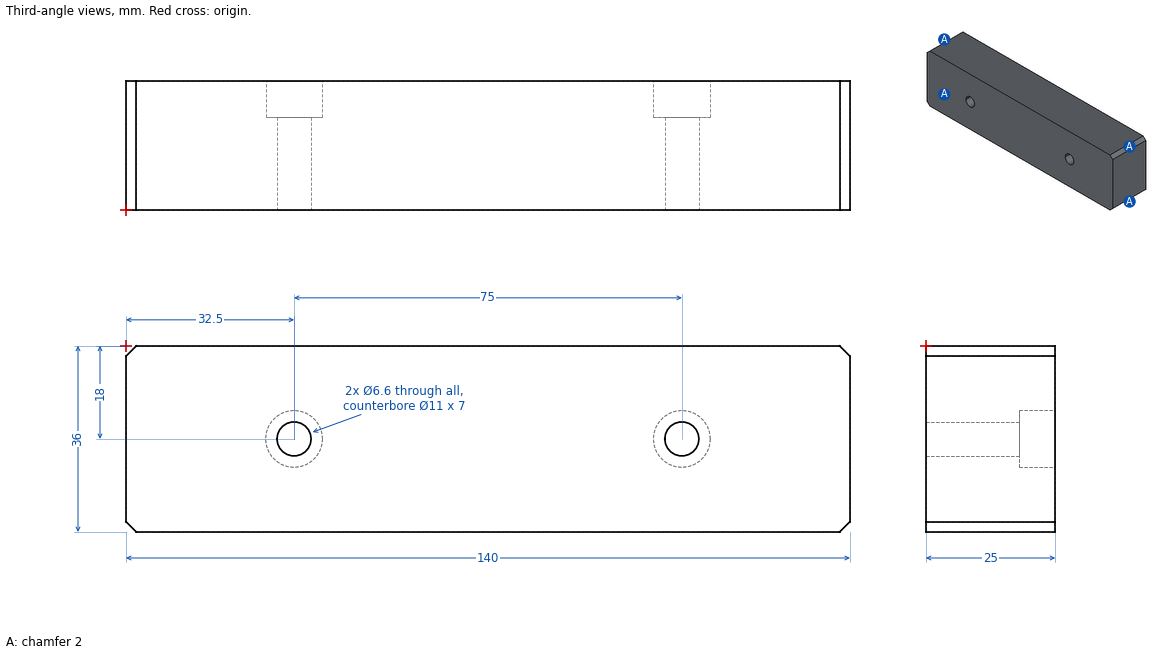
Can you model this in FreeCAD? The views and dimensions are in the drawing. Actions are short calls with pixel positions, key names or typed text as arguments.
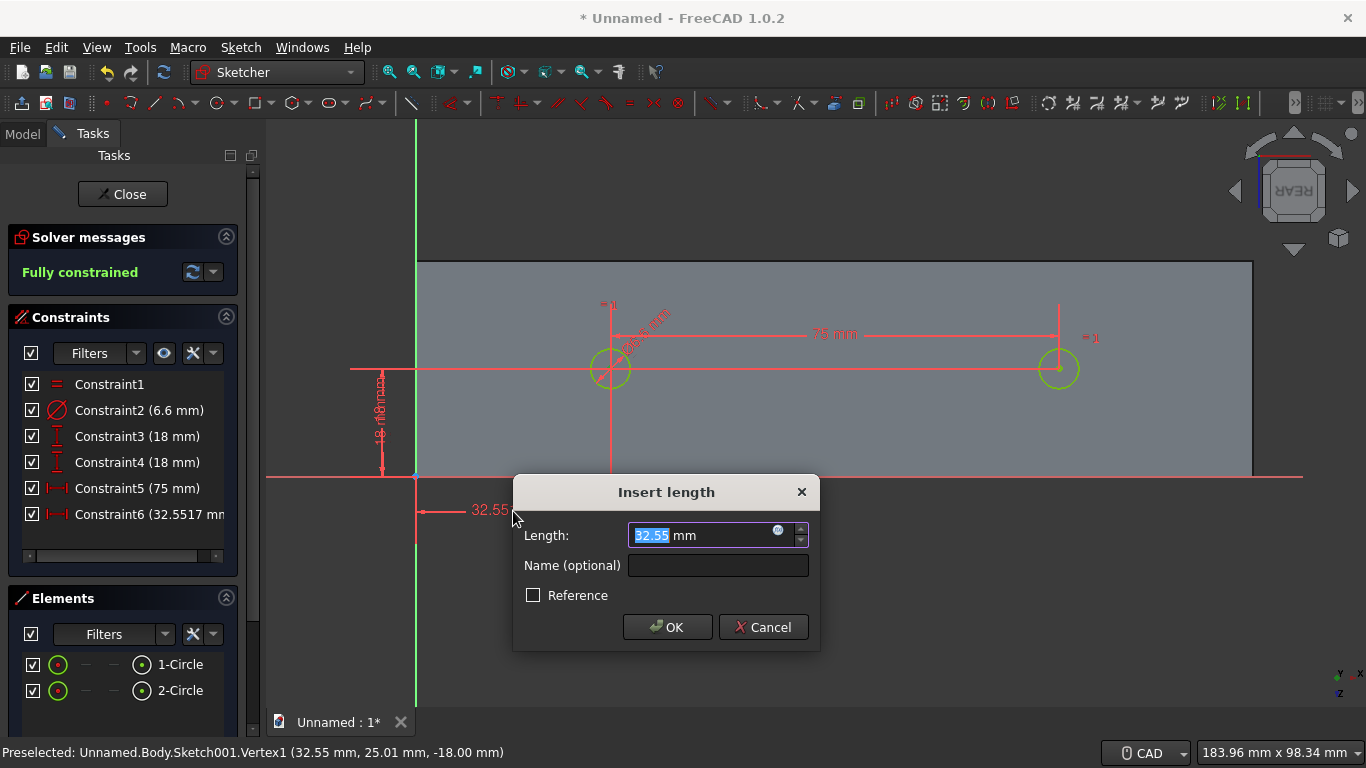
text(32.5)
key(Return)
key(Escape)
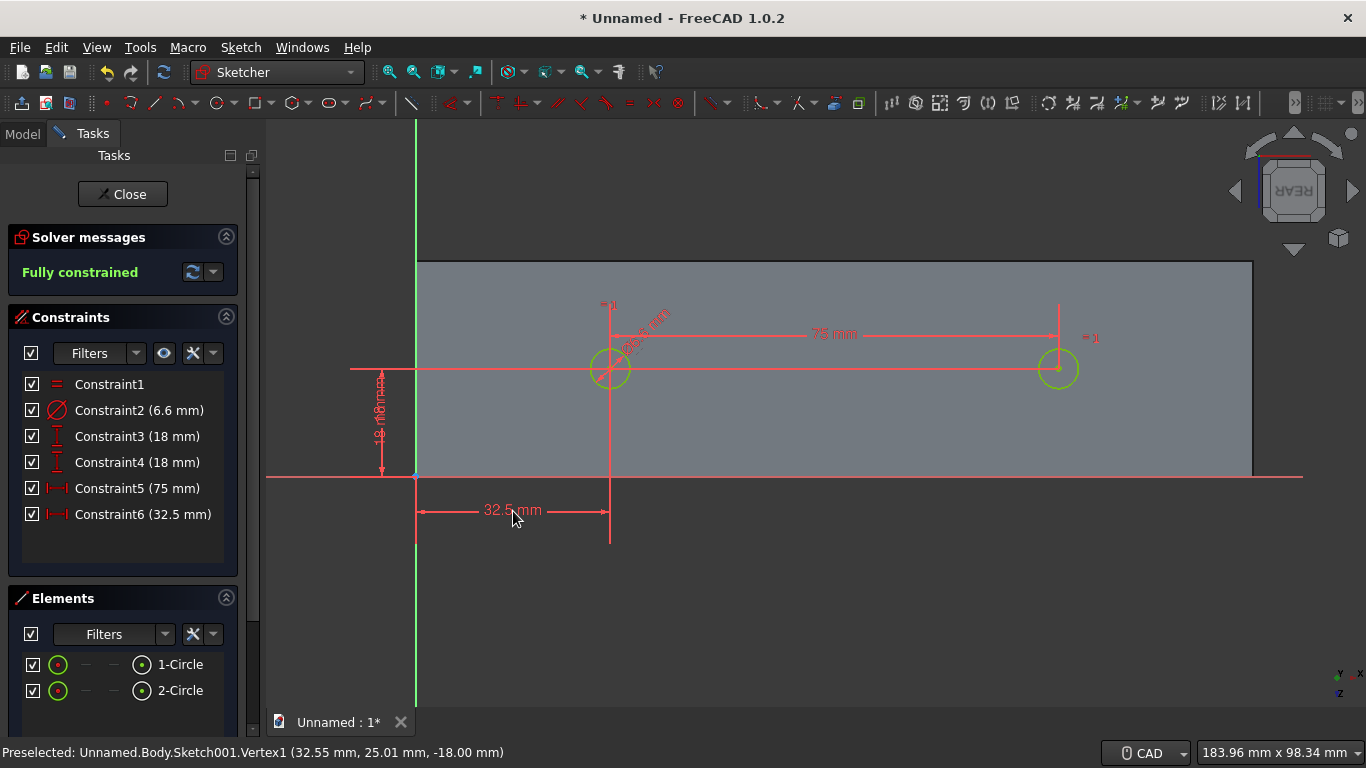
click(123, 194)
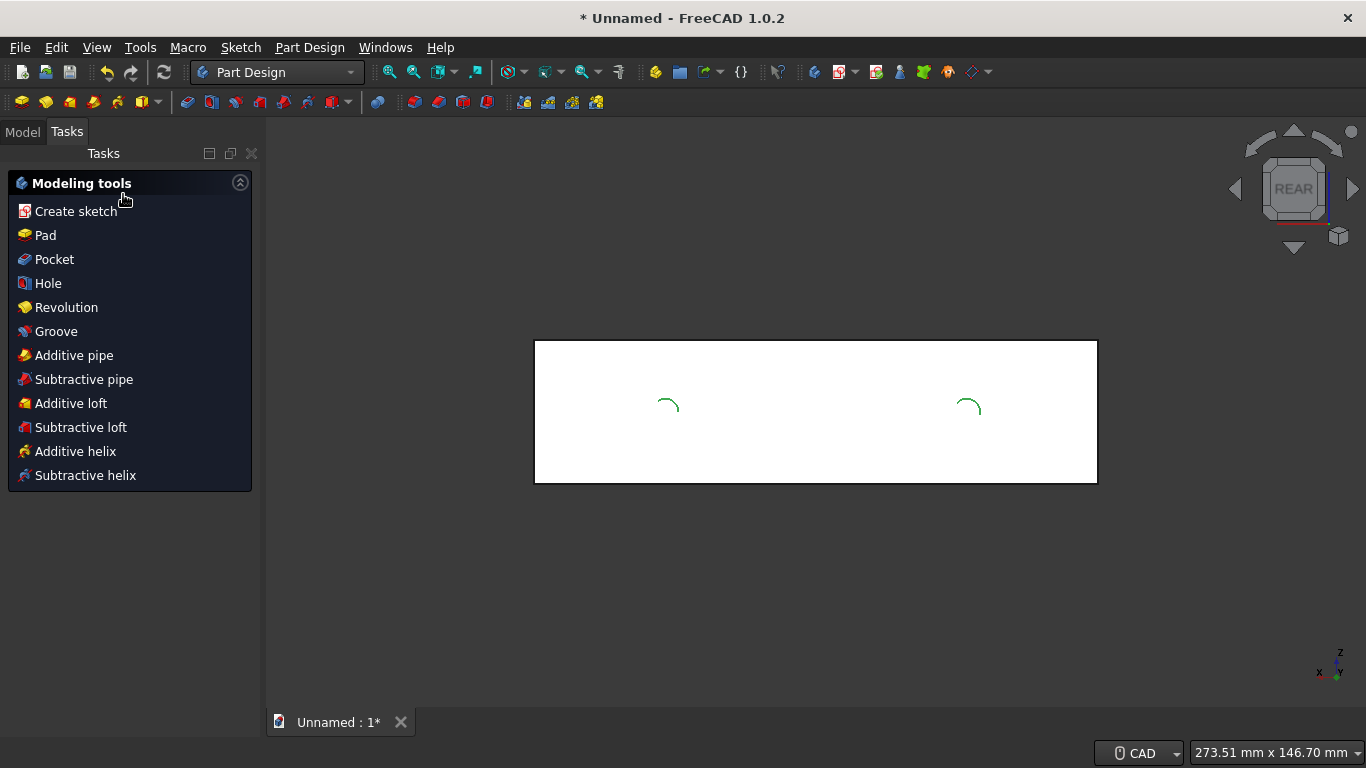
click(212, 102)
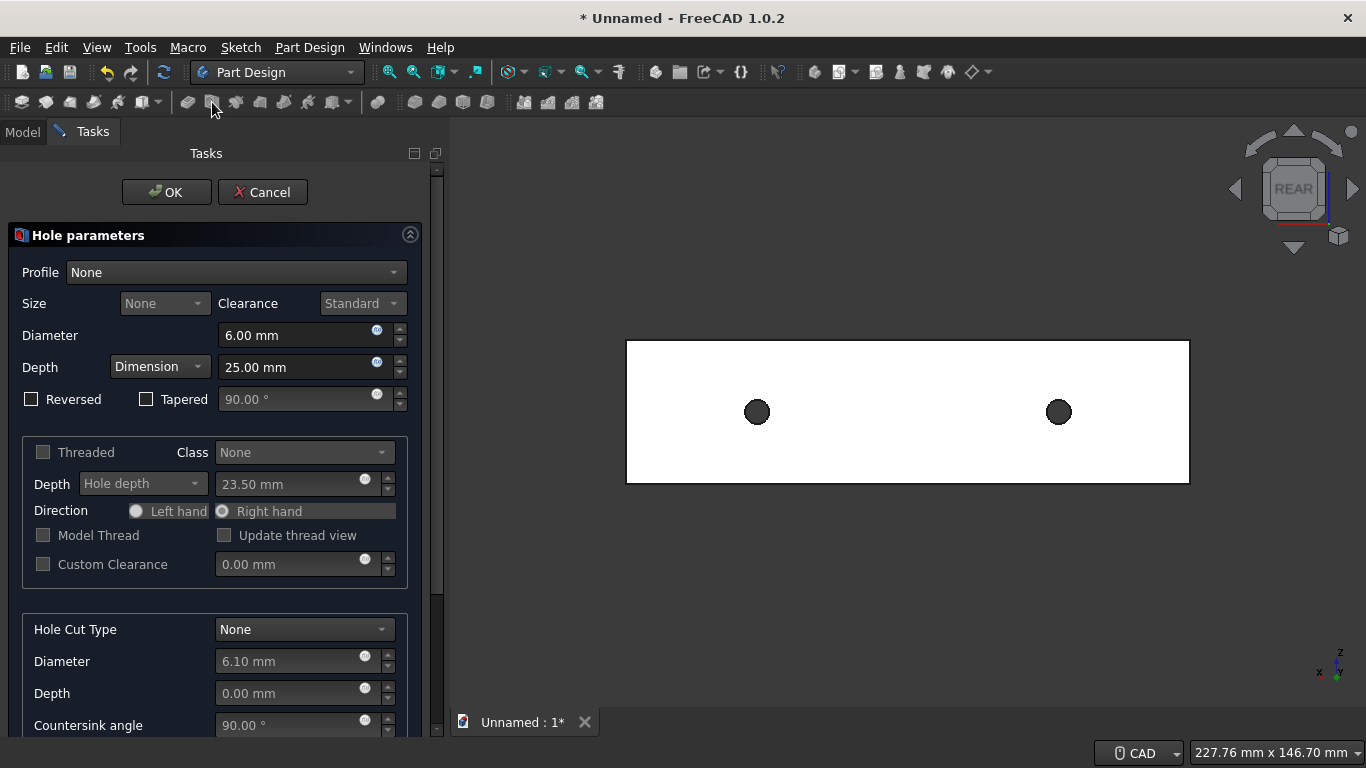
triple_click(305, 335)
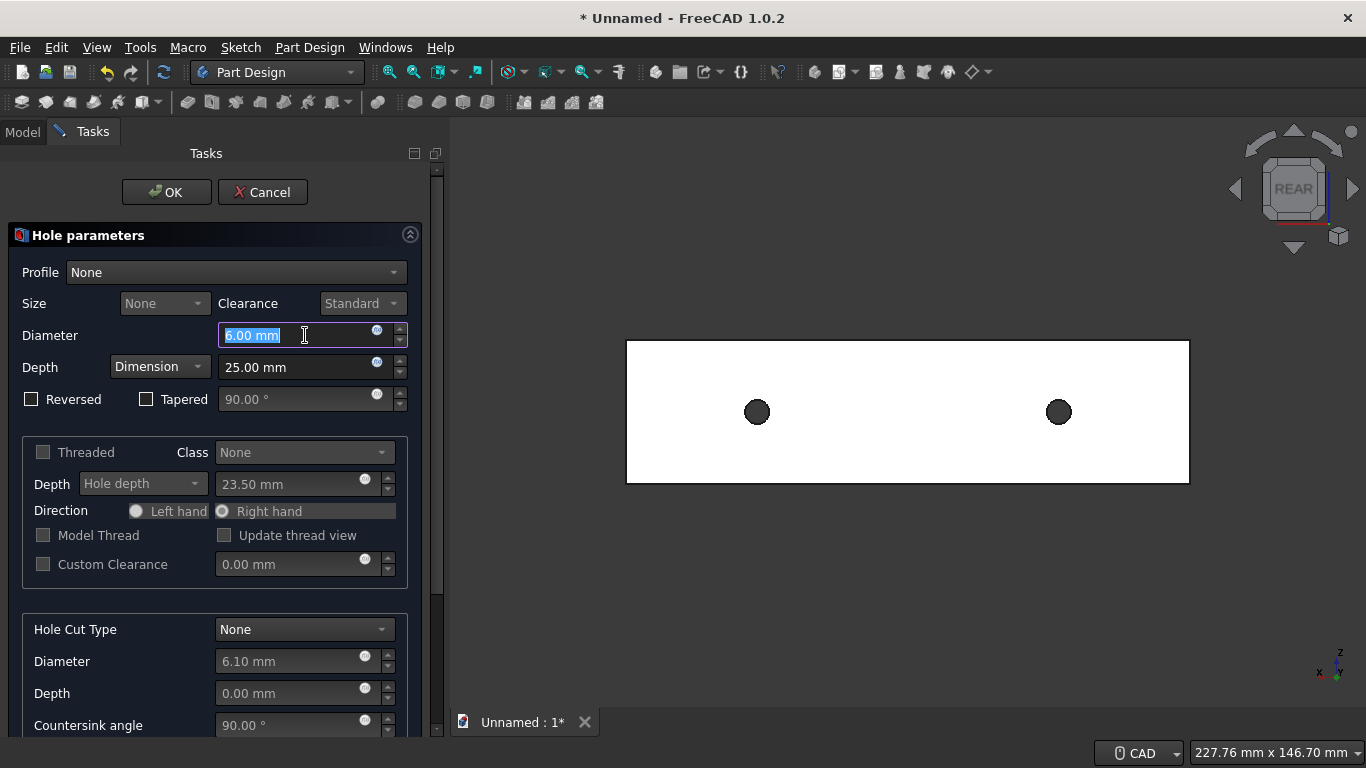
text(6.6)
key(Tab)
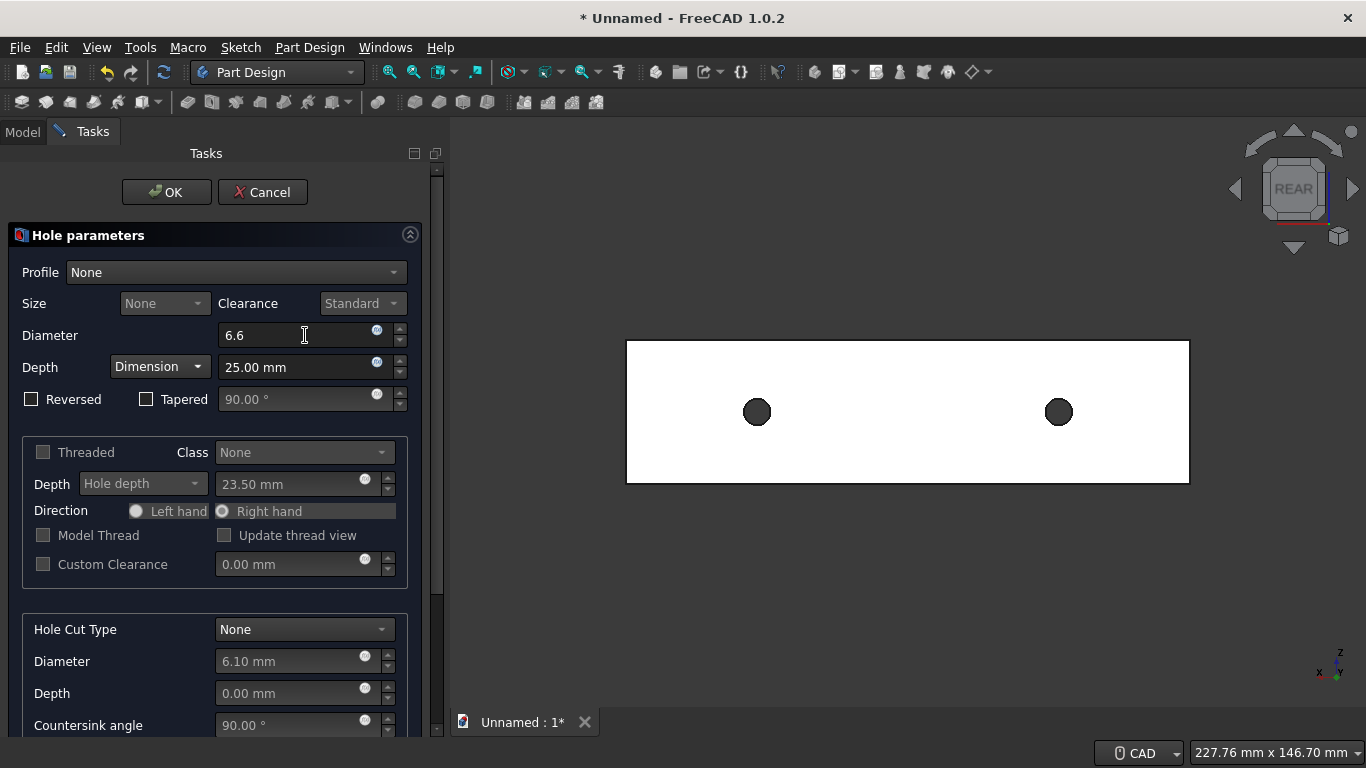
click(161, 366)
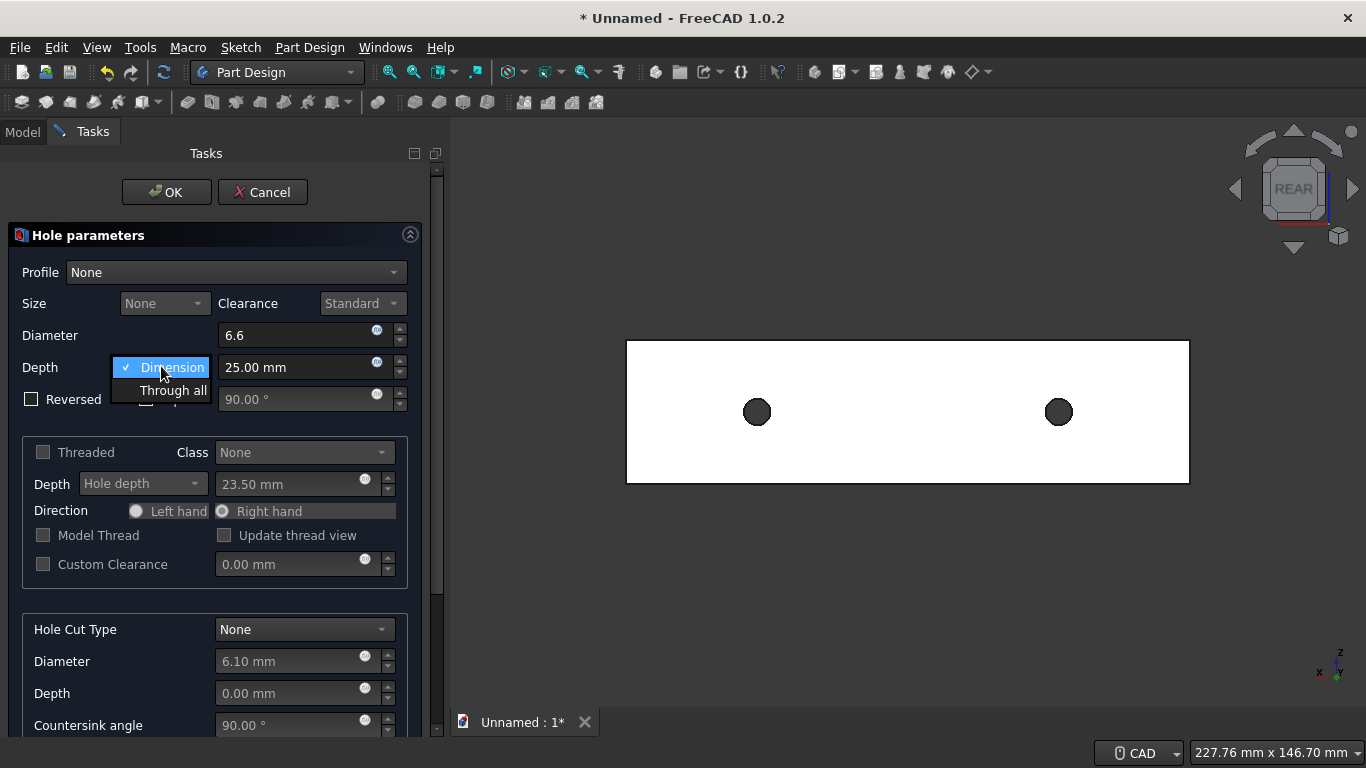
click(160, 390)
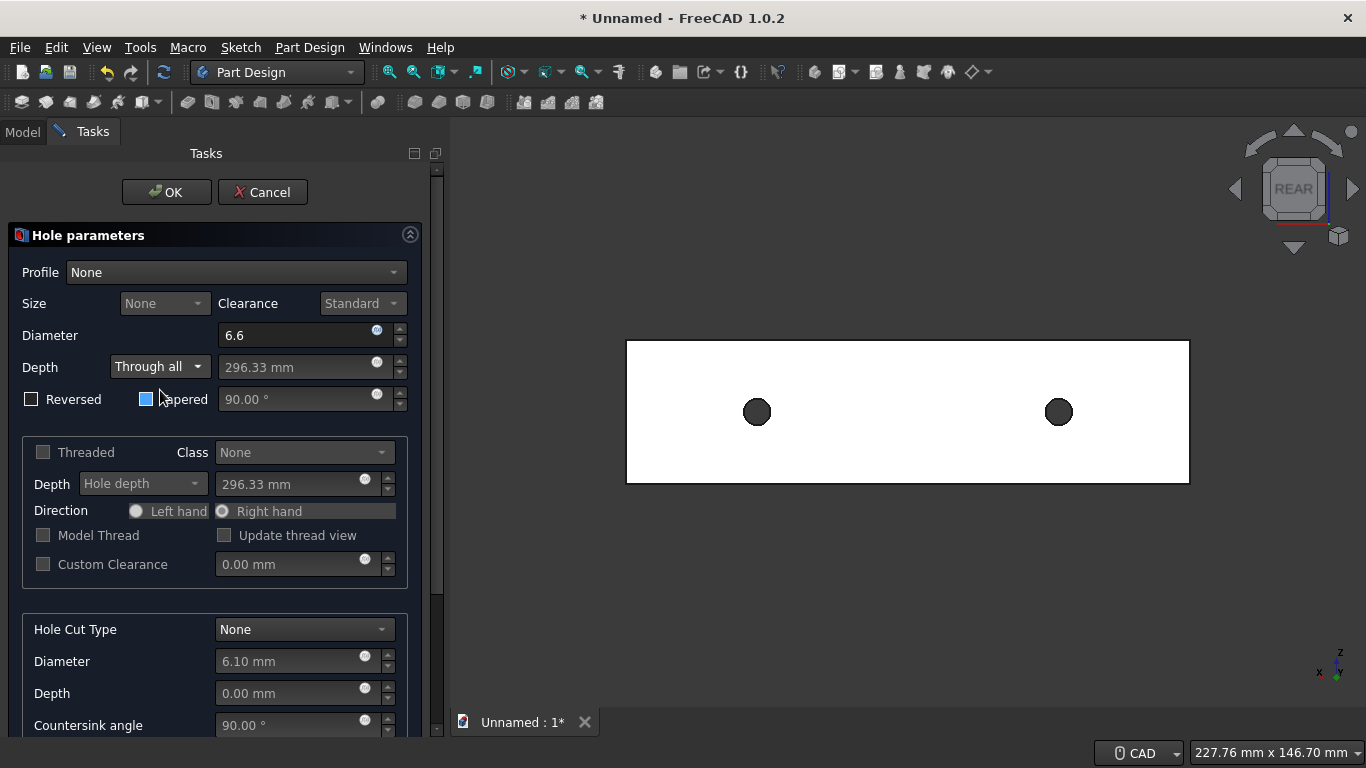
click(306, 630)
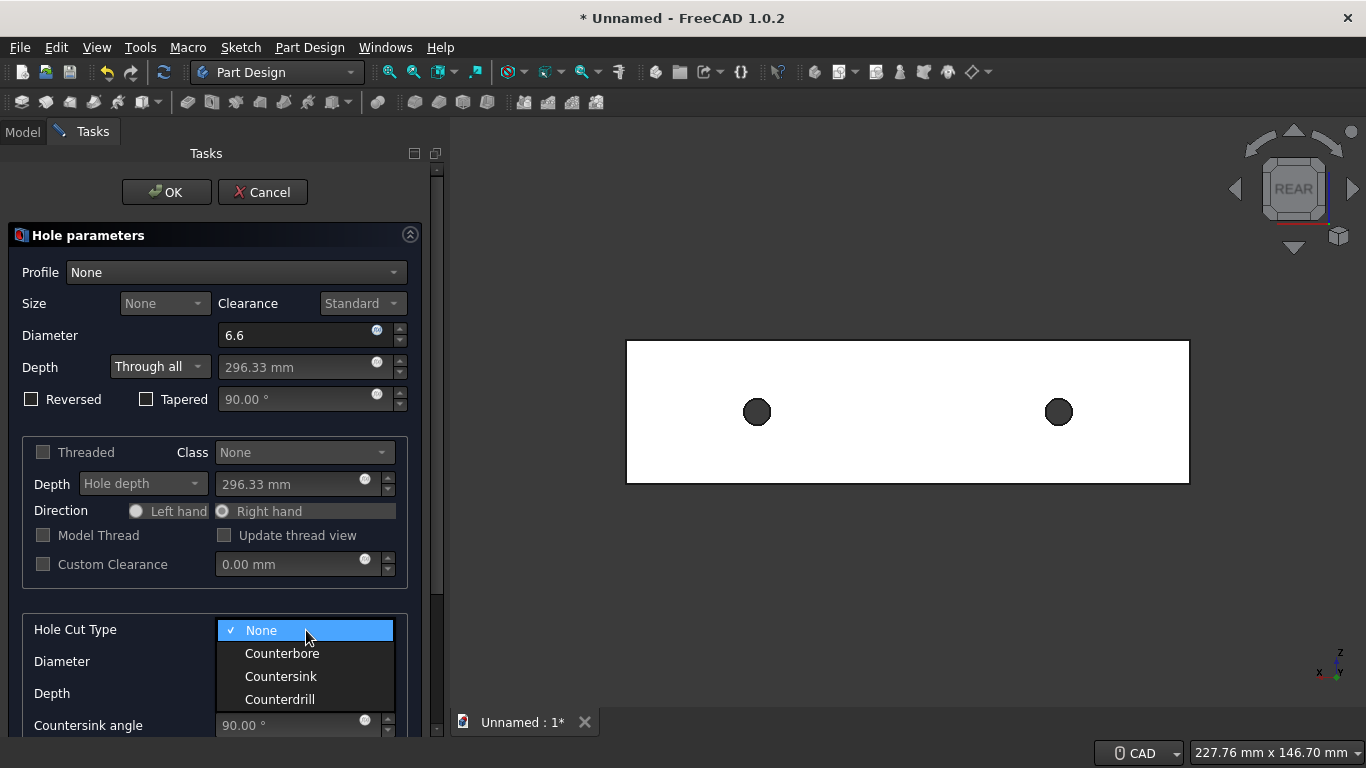
click(304, 654)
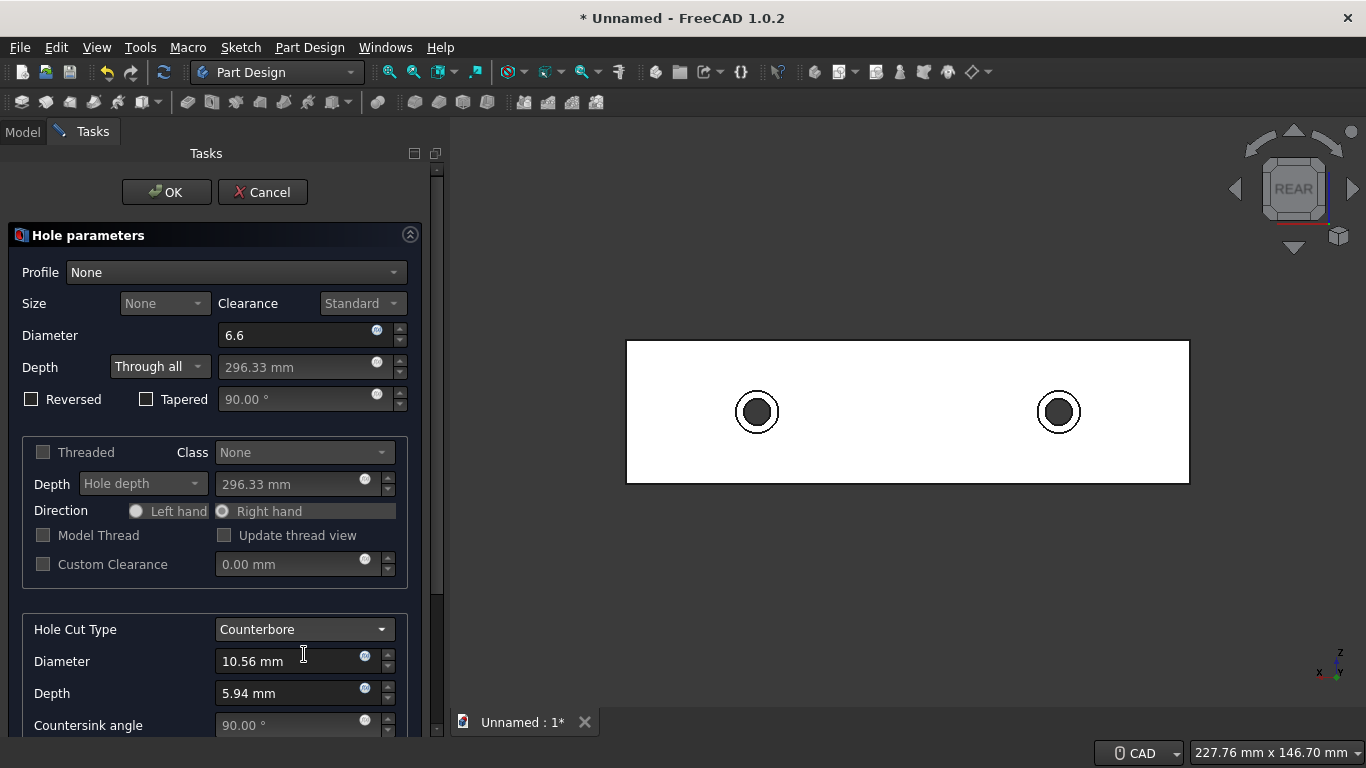
triple_click(298, 661)